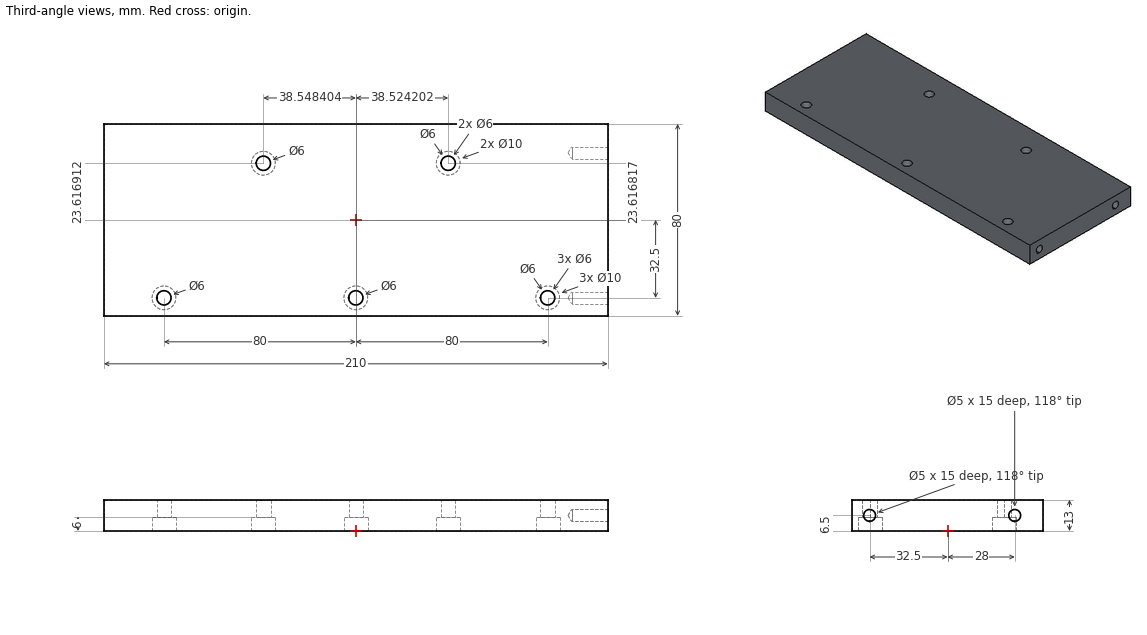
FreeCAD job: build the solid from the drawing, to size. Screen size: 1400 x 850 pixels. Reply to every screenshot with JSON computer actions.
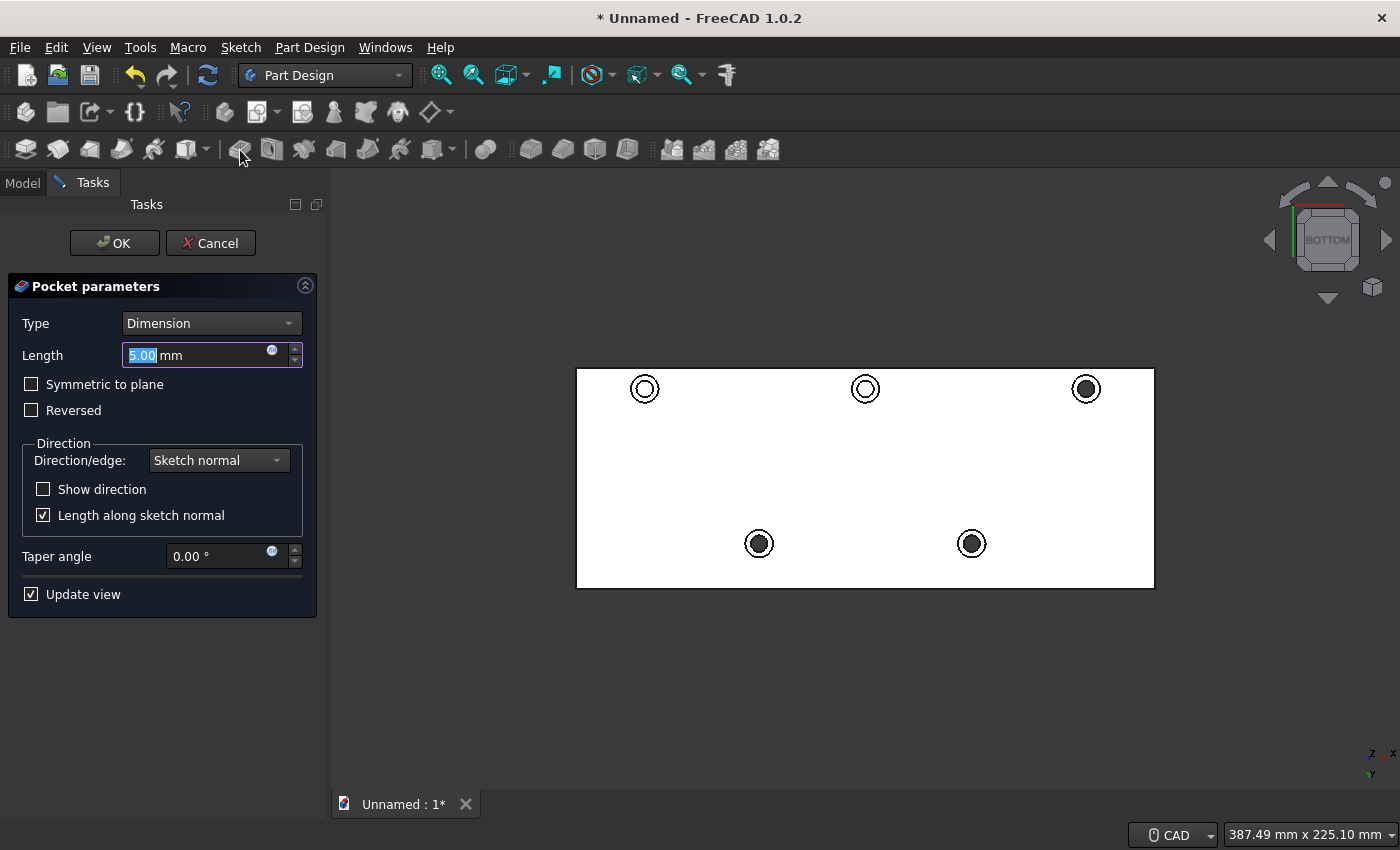
{"action": "left_click", "coordinate": [212, 324]}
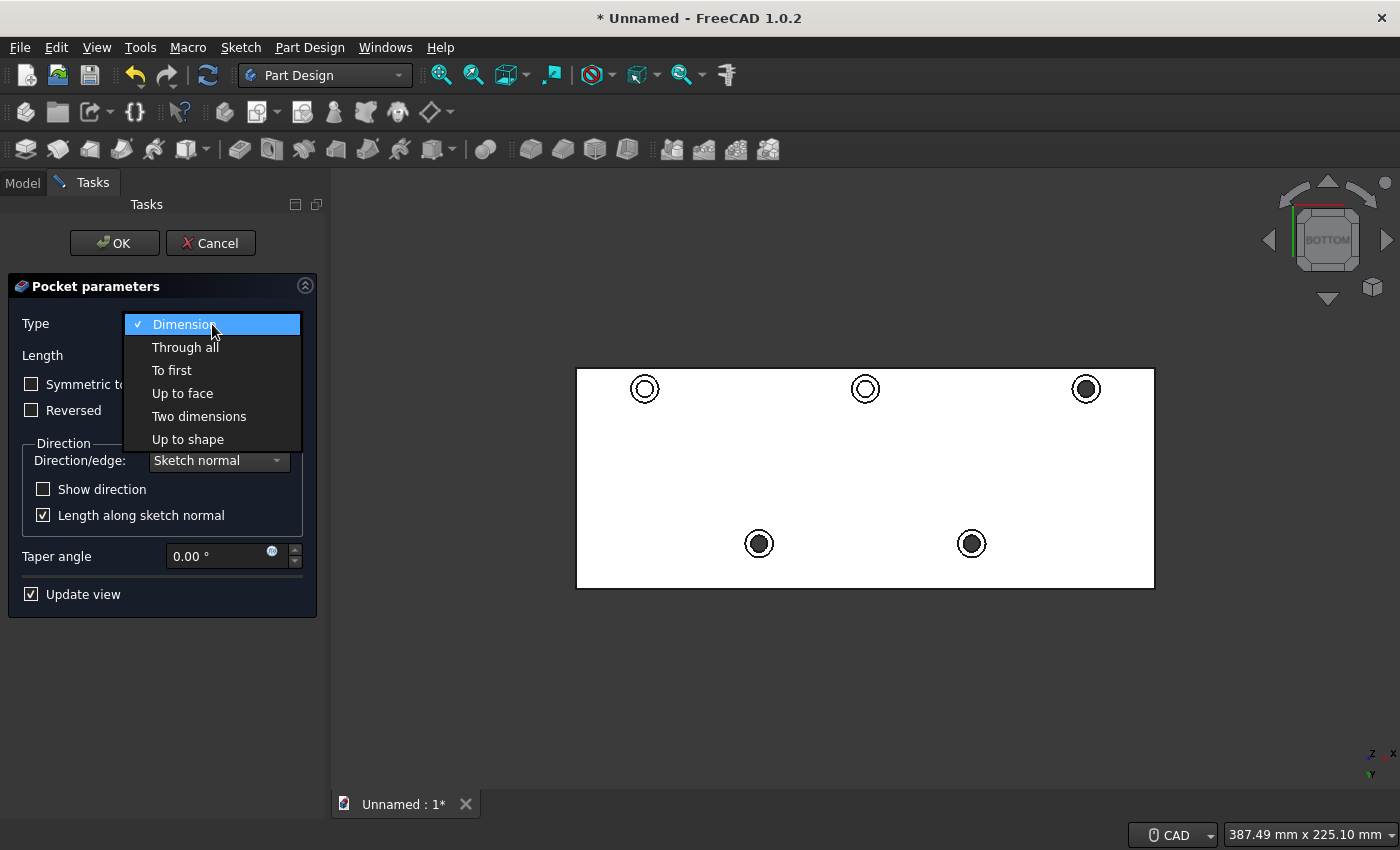
{"action": "left_click", "coordinate": [212, 370]}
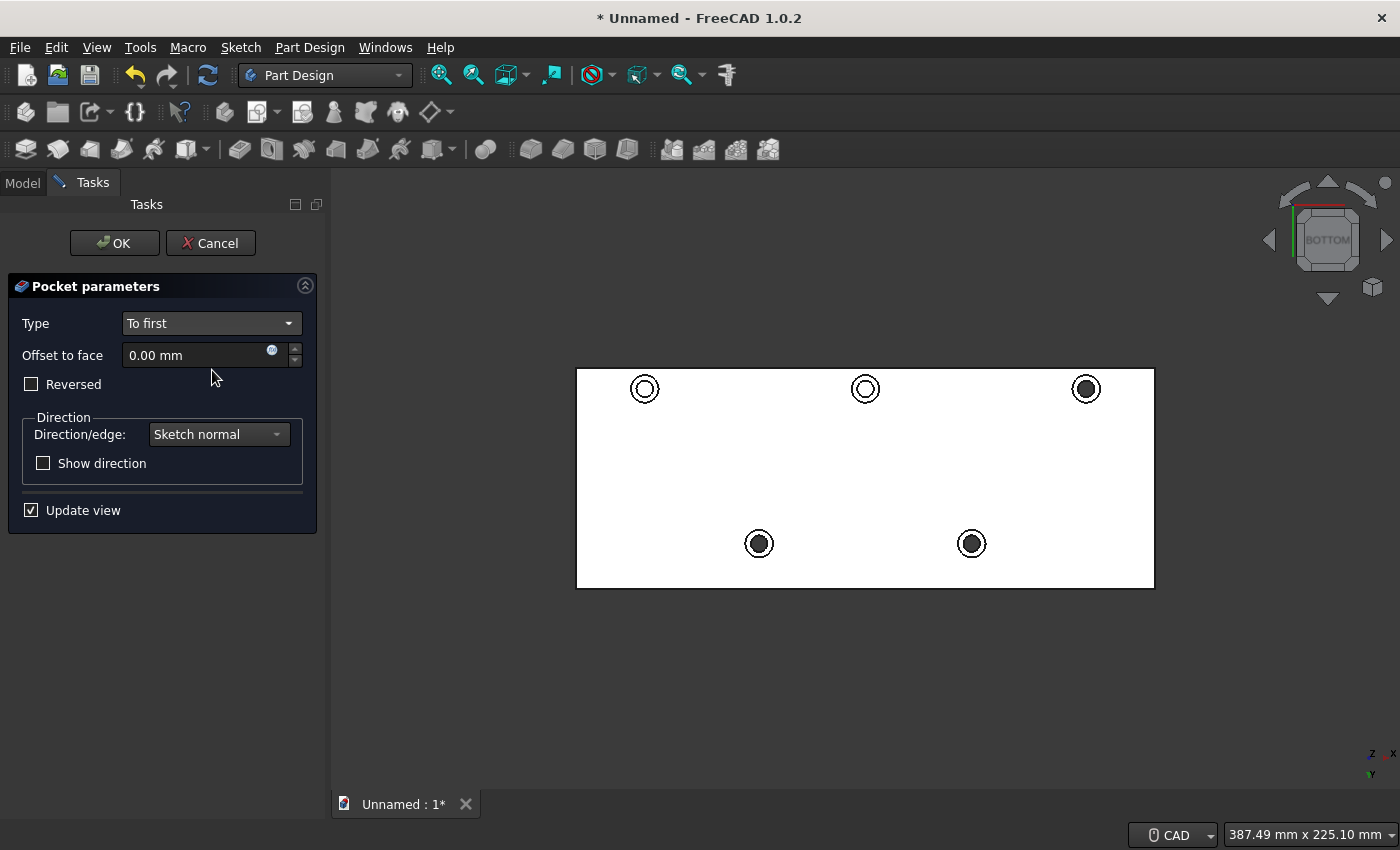
{"action": "left_click", "coordinate": [30, 384]}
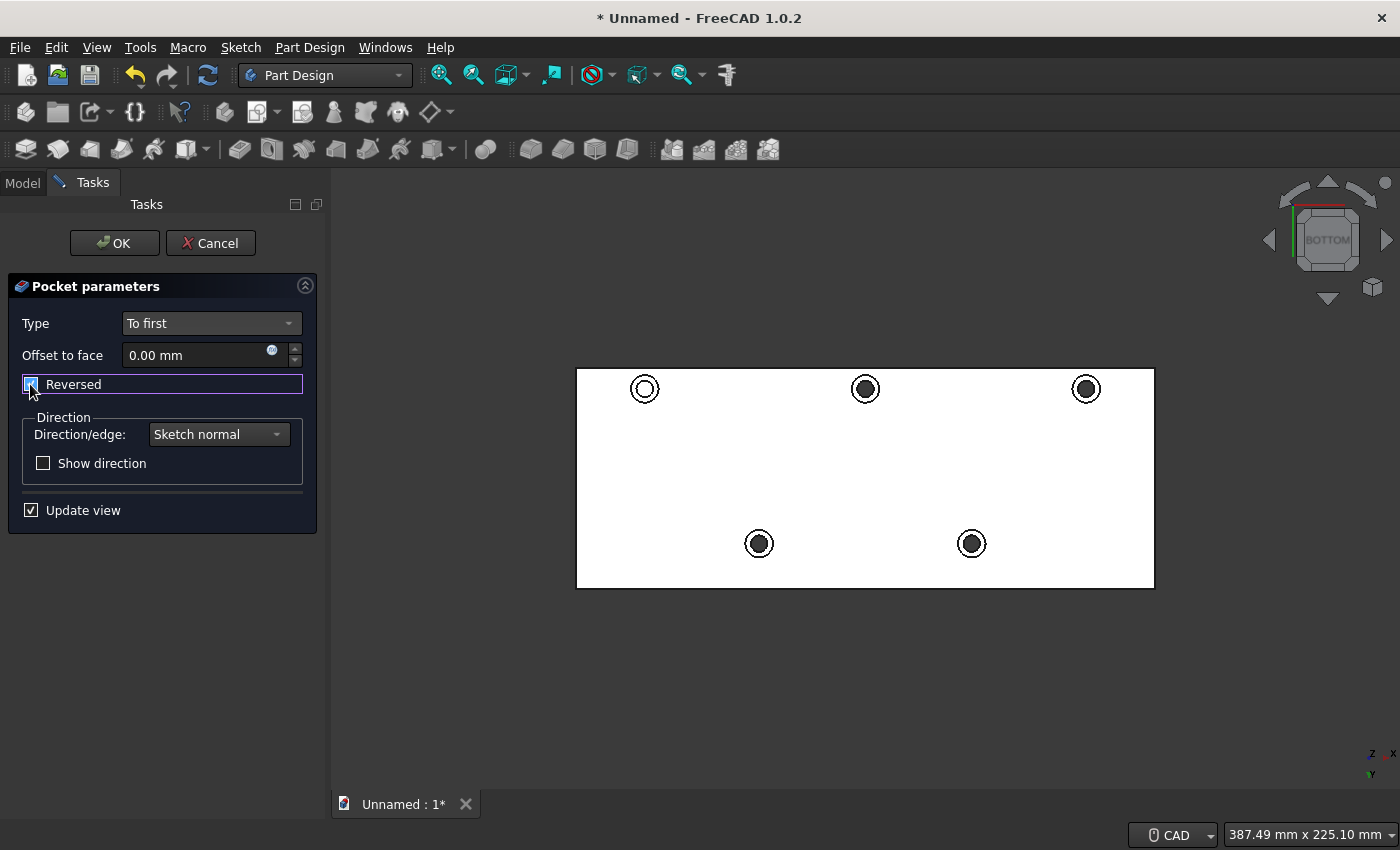
{"action": "left_click", "coordinate": [115, 243]}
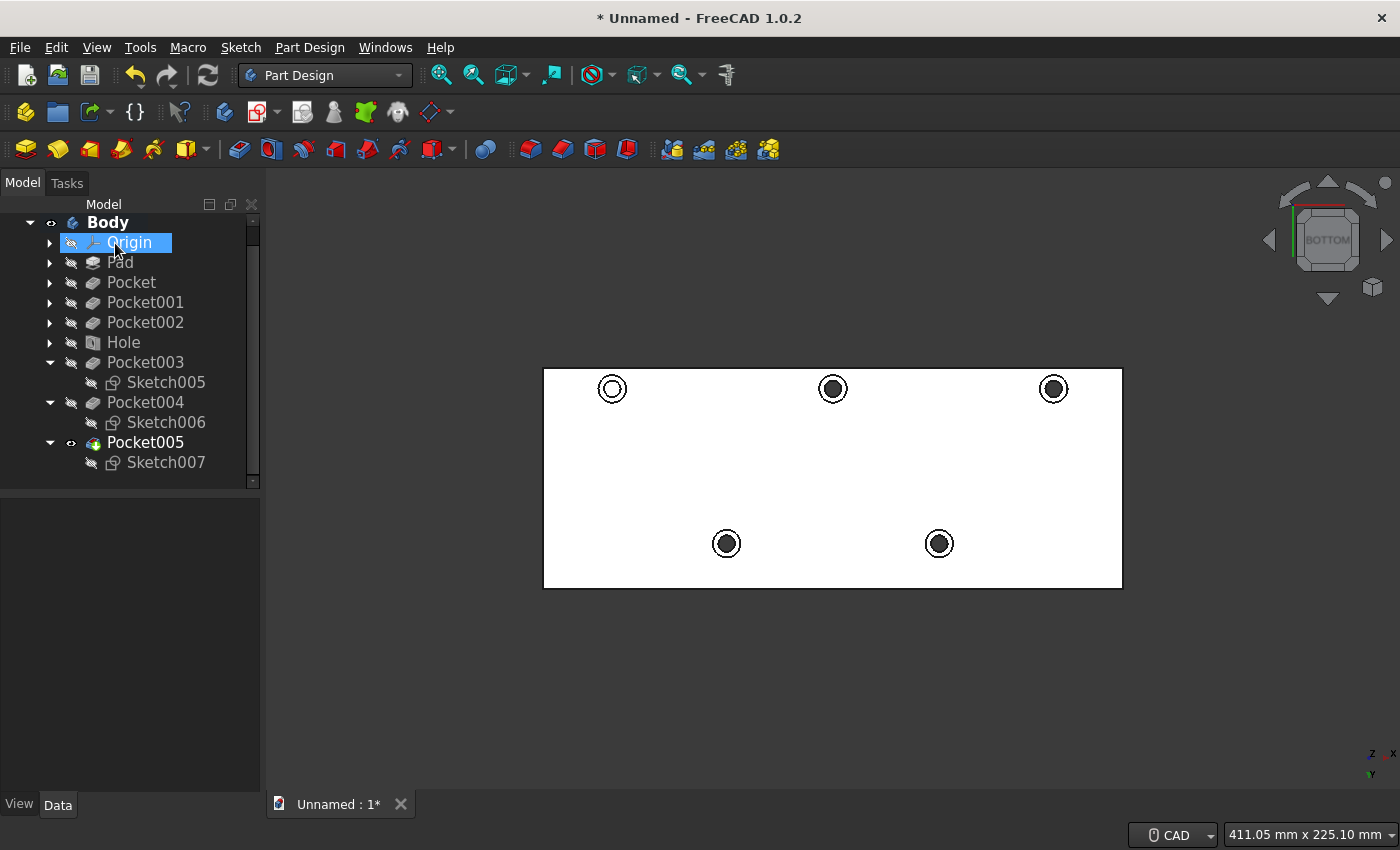
{"action": "left_click", "coordinate": [258, 112]}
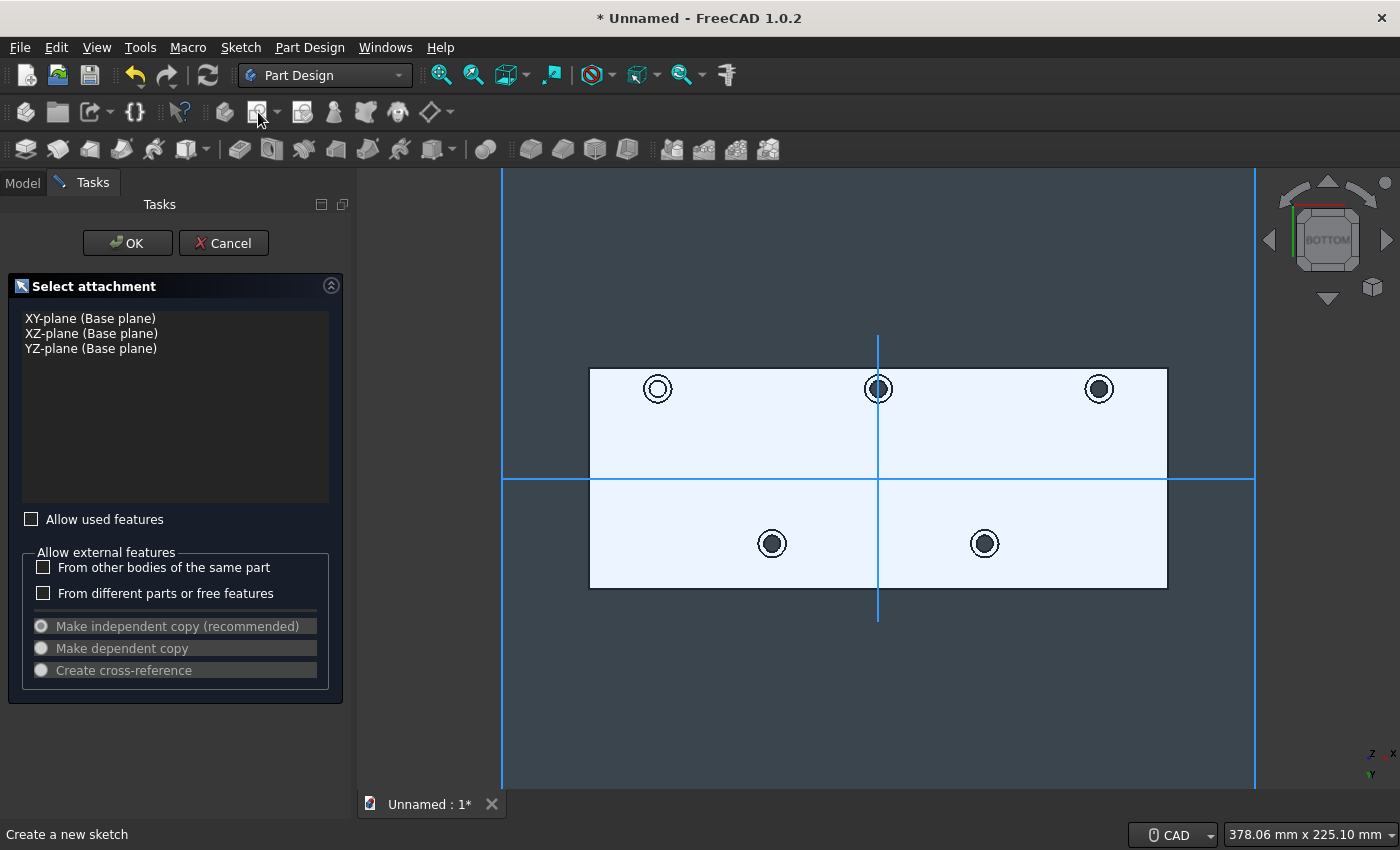
{"action": "left_click", "coordinate": [82, 318]}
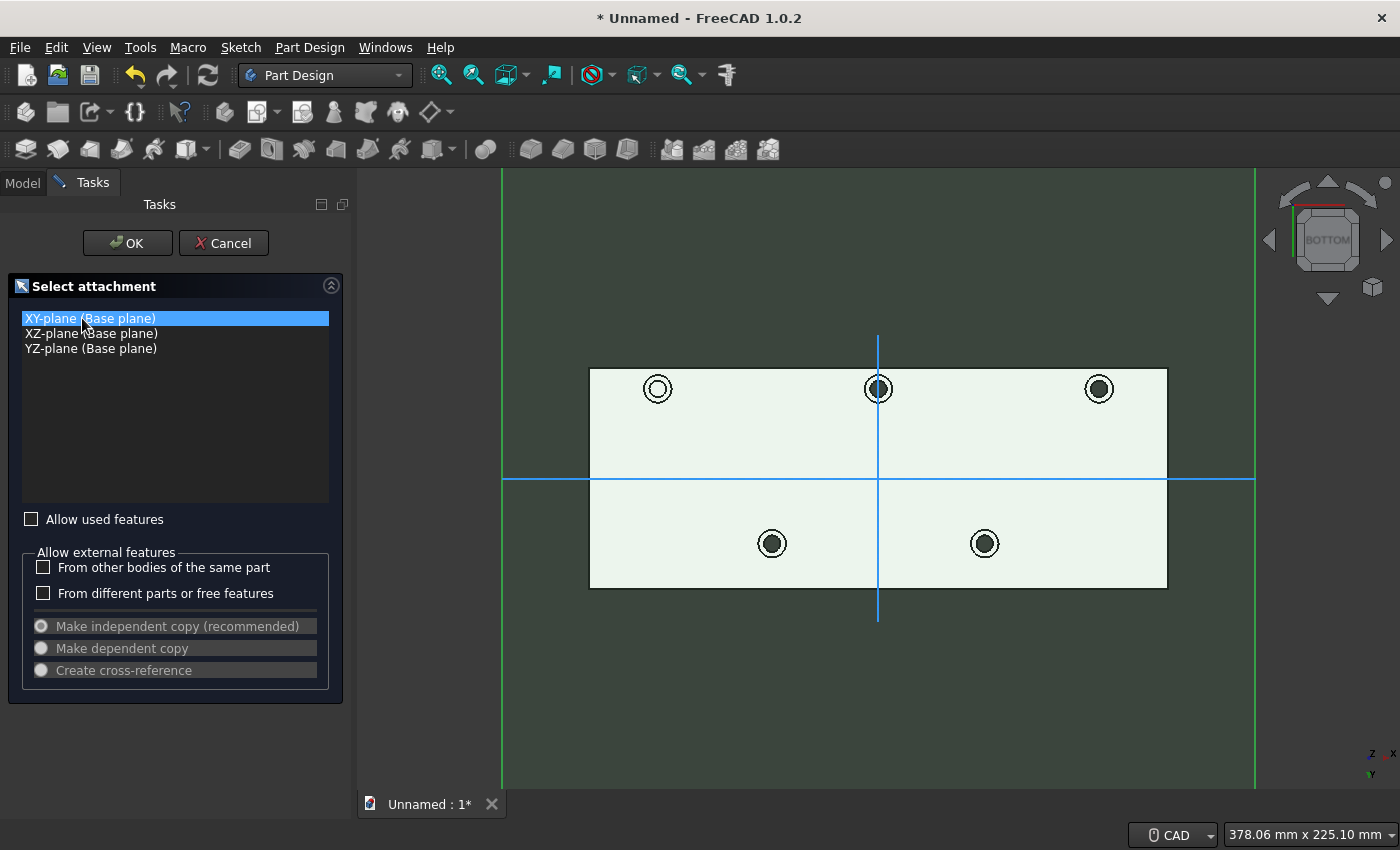
{"action": "left_click", "coordinate": [128, 243]}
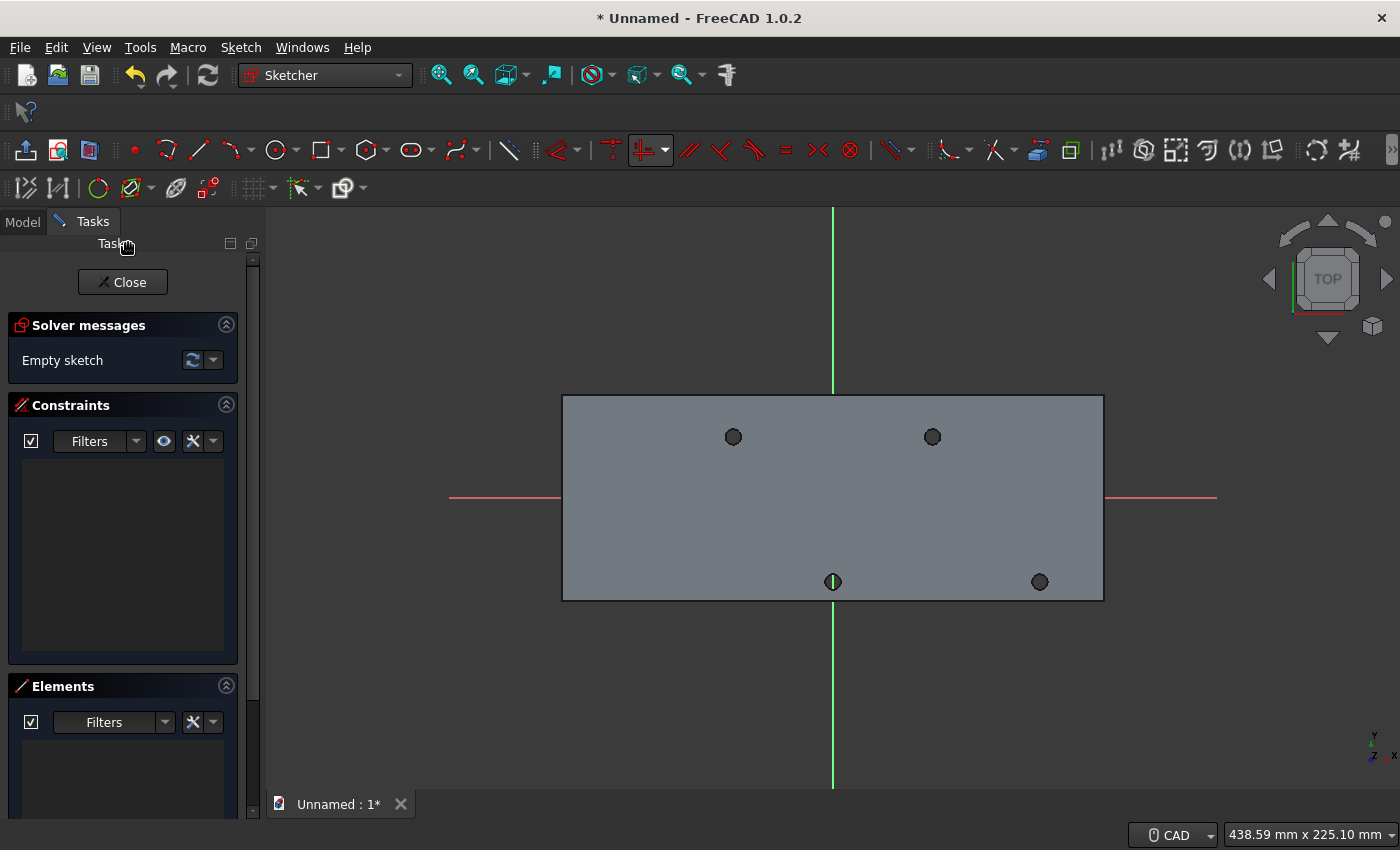
{"action": "key", "text": "q s"}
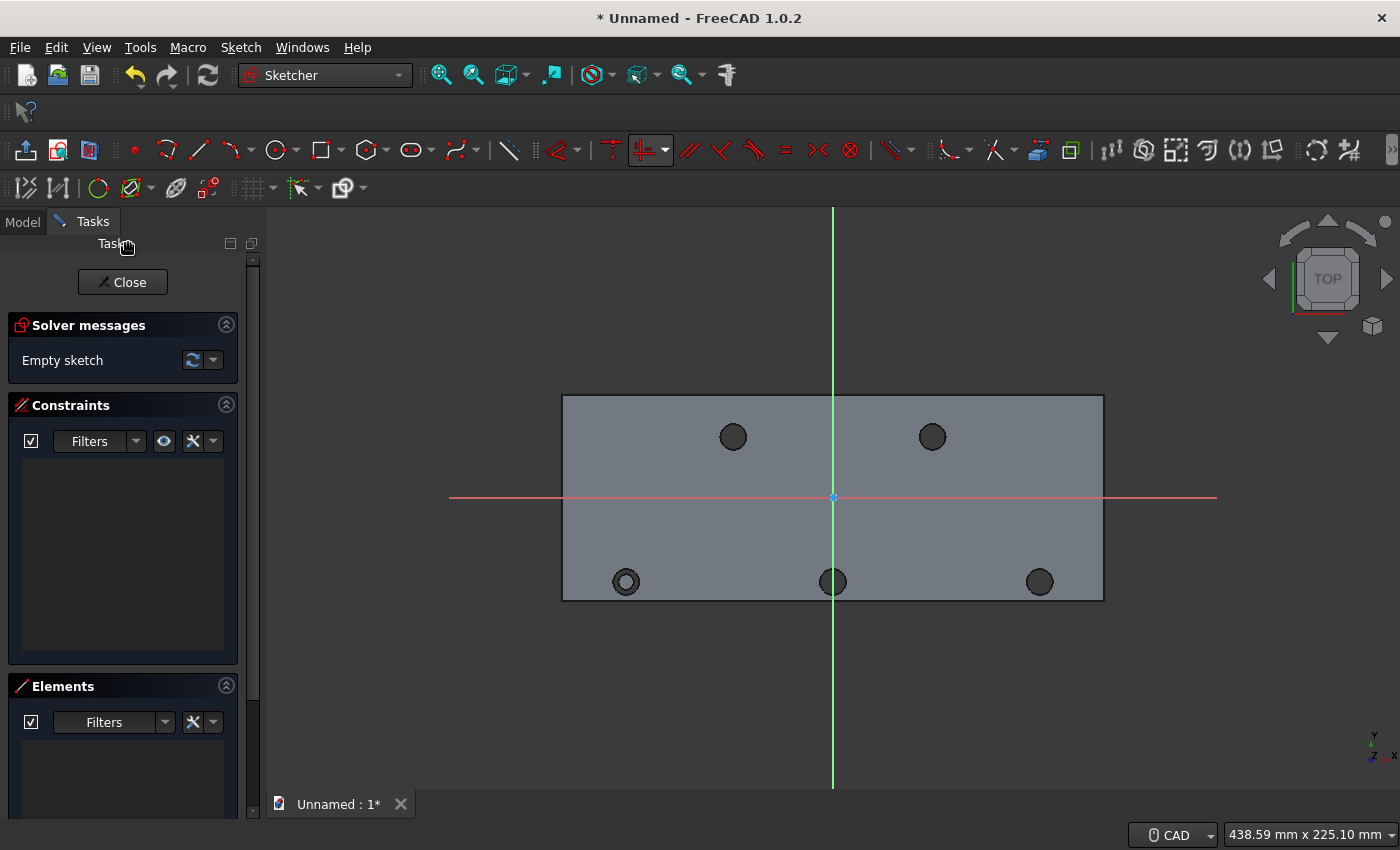
{"action": "scroll", "coordinate": [619, 586], "scroll_direction": "up", "scroll_amount": 15}